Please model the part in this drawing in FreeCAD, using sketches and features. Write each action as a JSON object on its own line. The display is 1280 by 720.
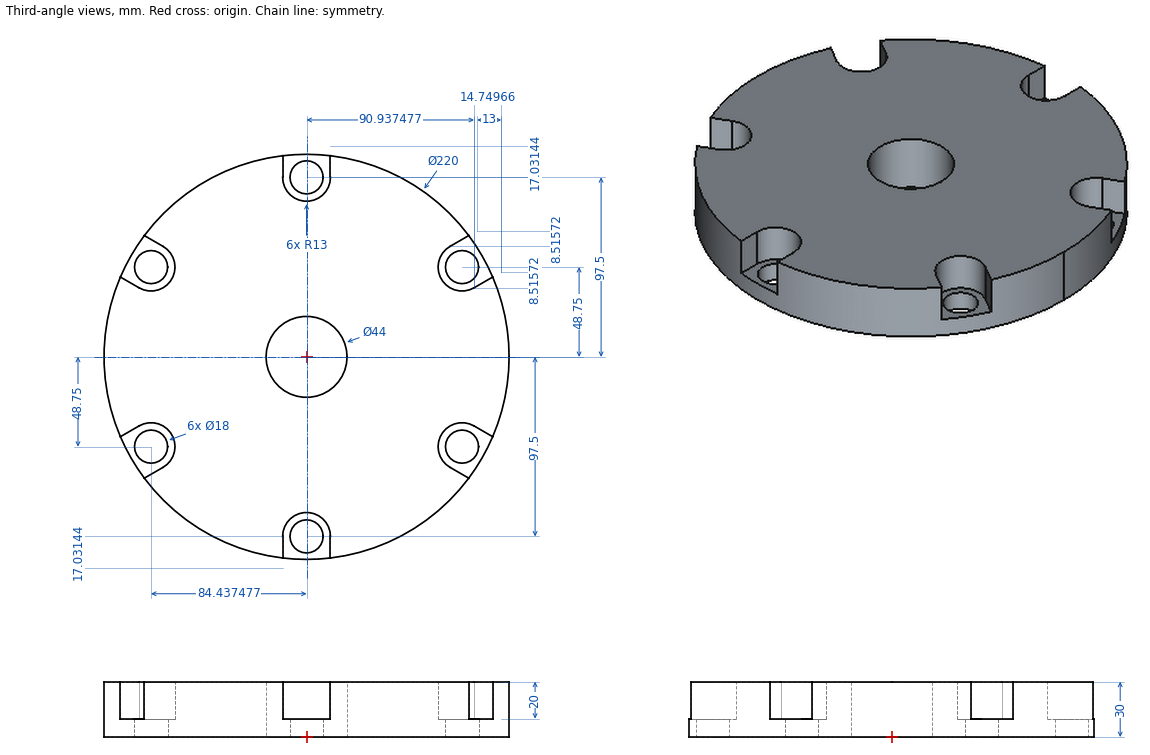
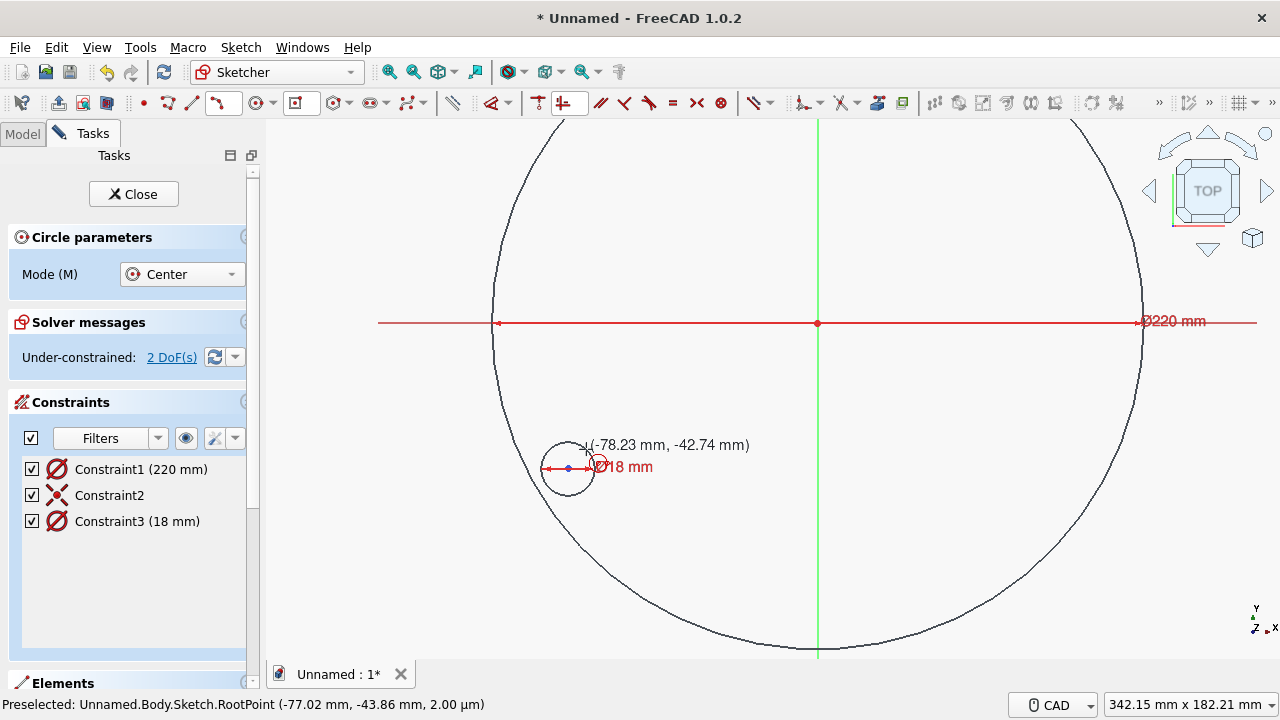
{"action": "left_click", "coordinate": [818, 612]}
{"action": "mouse_move", "coordinate": [837, 593]}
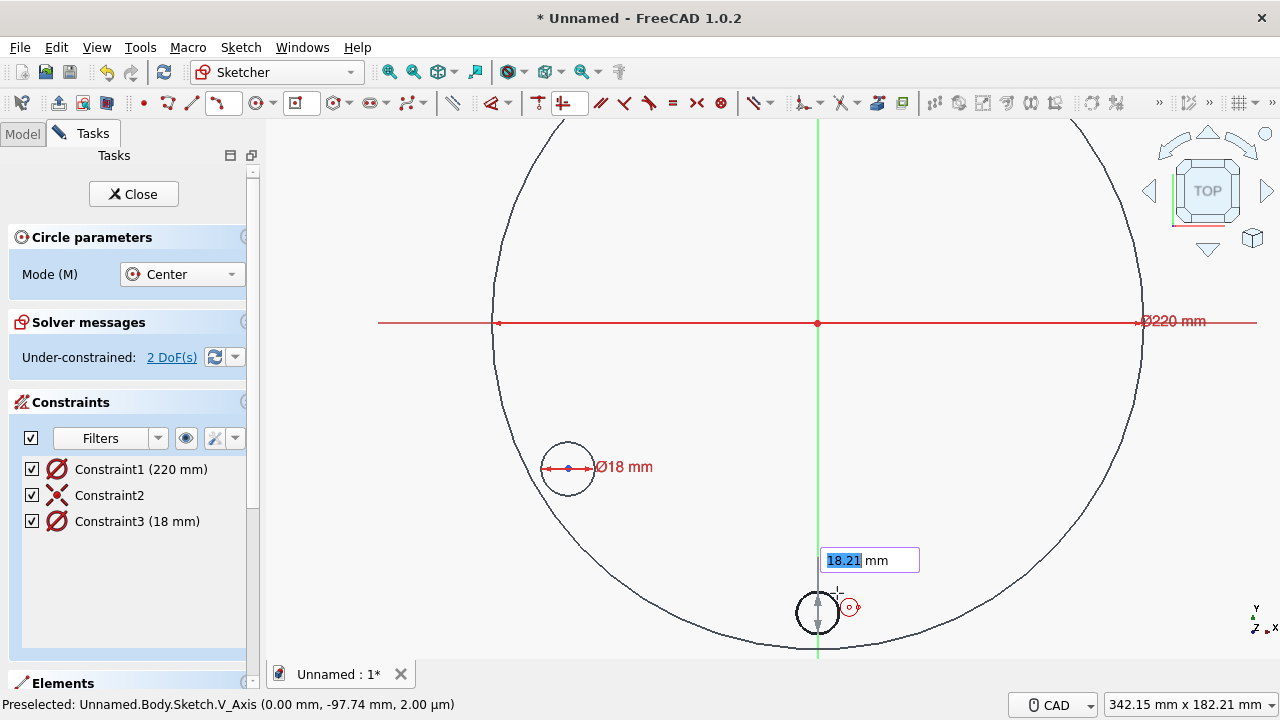
{"action": "type", "text": "18"}
{"action": "key", "text": "Return"}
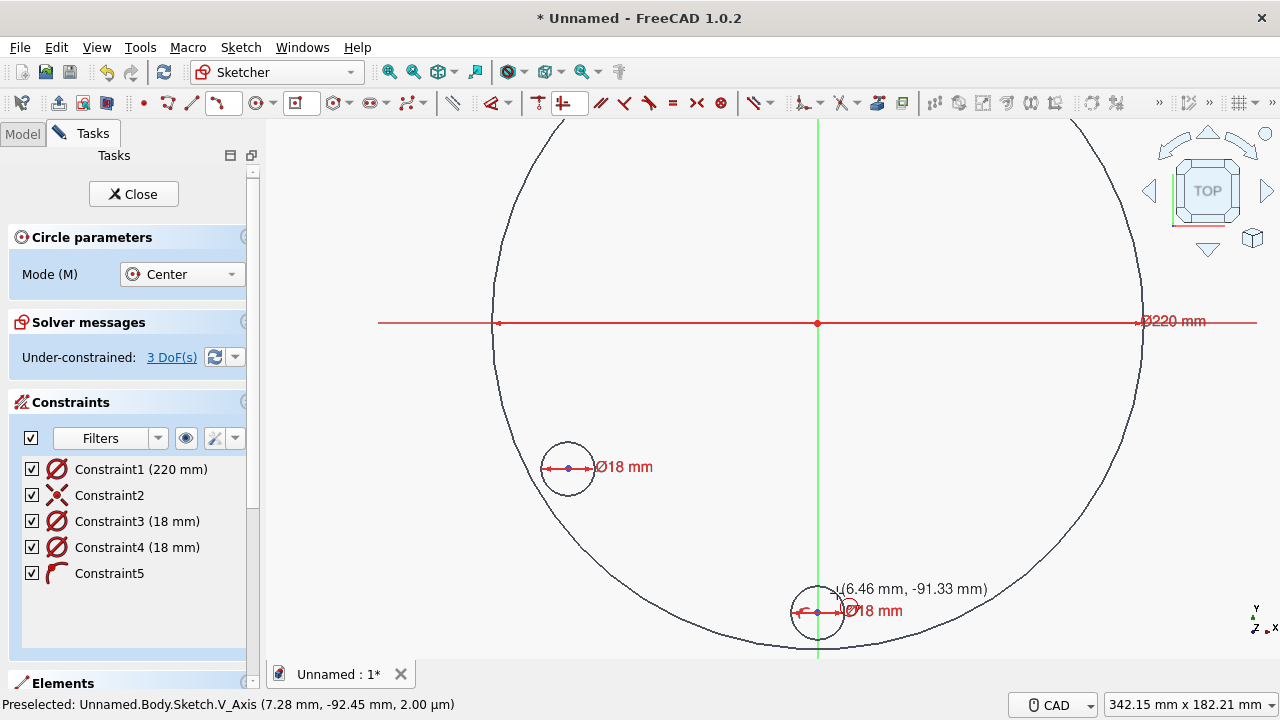
{"action": "left_click", "coordinate": [1068, 468]}
{"action": "mouse_move", "coordinate": [1087, 449]}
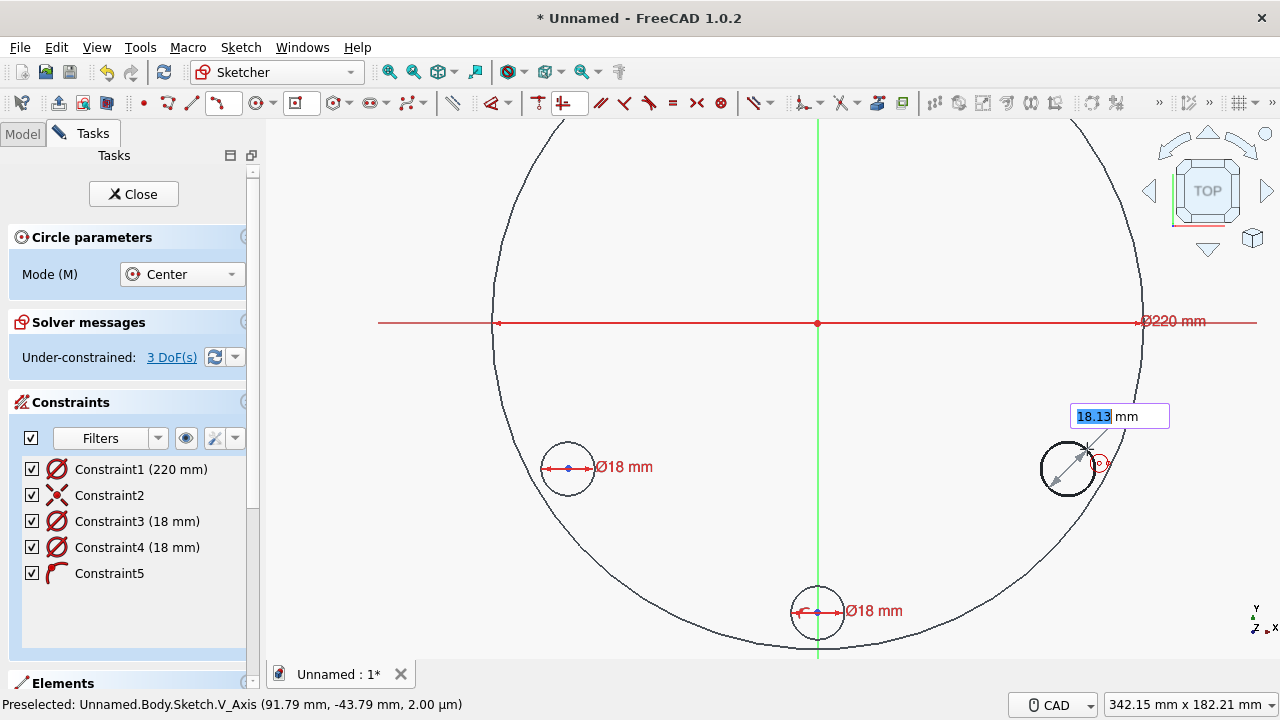
{"action": "type", "text": "18"}
{"action": "key", "text": "Return"}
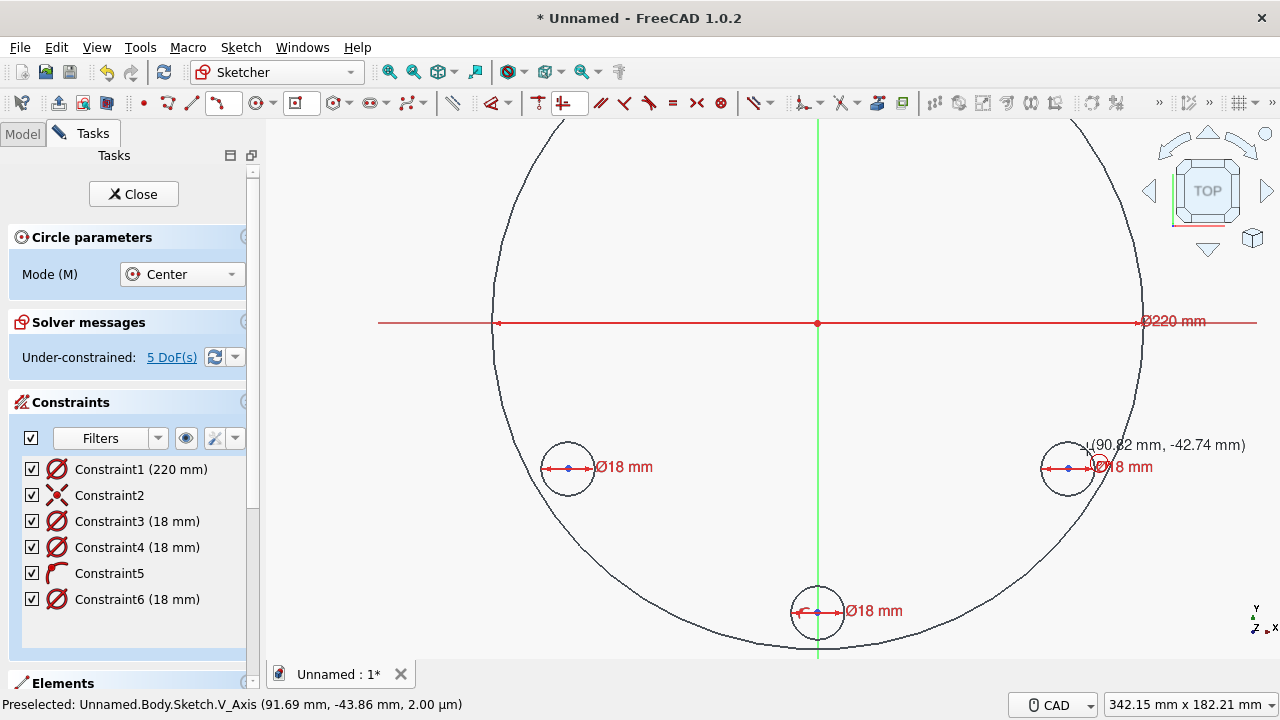
{"action": "left_click", "coordinate": [568, 179]}
{"action": "mouse_move", "coordinate": [586, 160]}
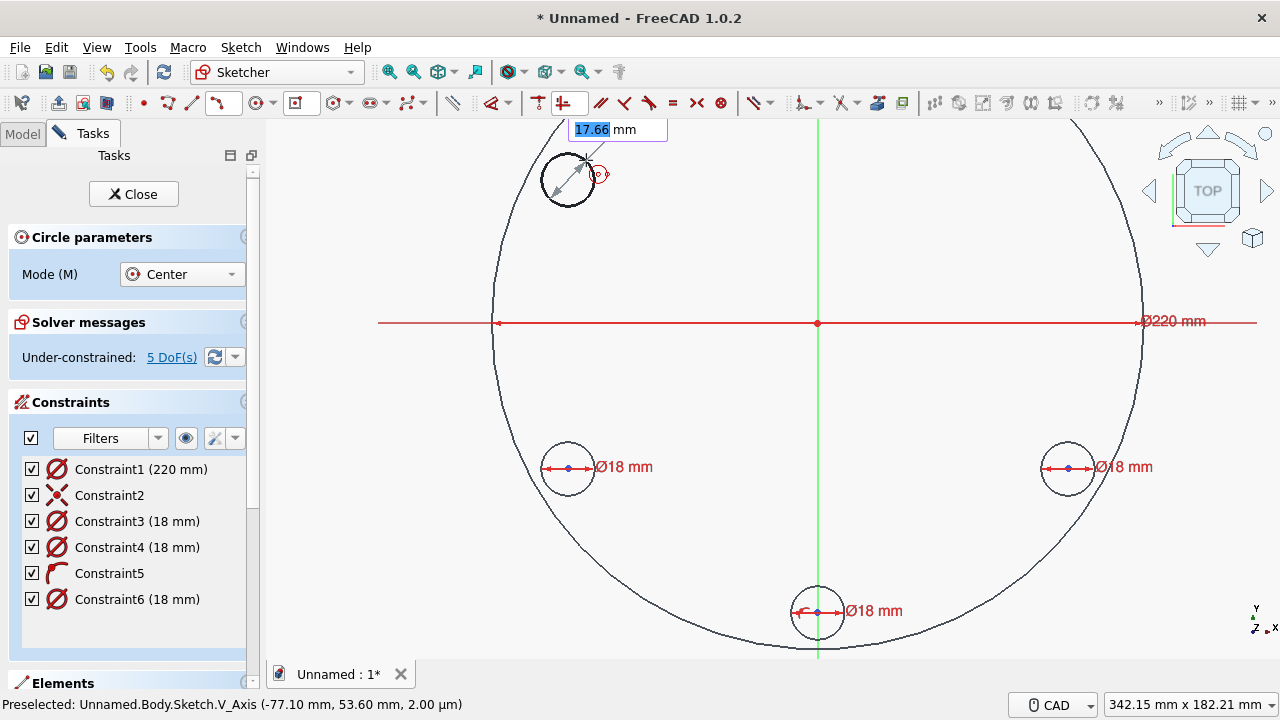
{"action": "type", "text": "18"}
{"action": "key", "text": "Return"}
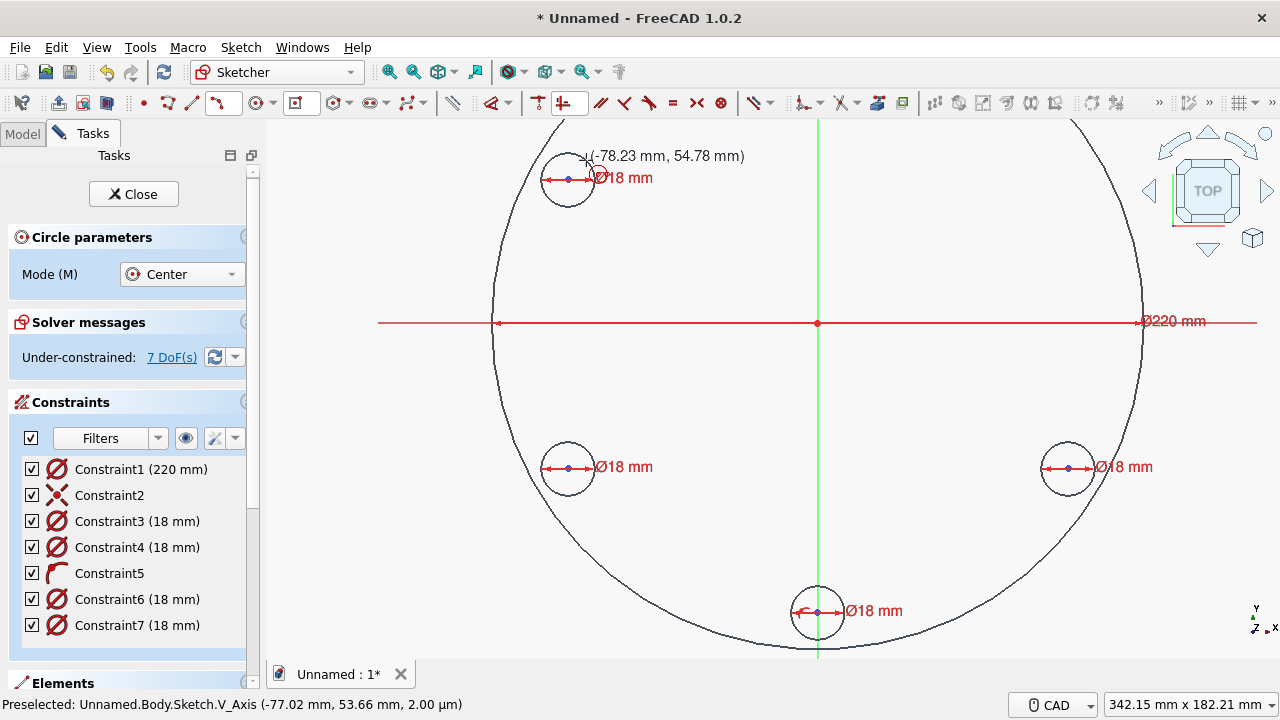
{"action": "left_click", "coordinate": [818, 323]}
{"action": "mouse_move", "coordinate": [864, 277]}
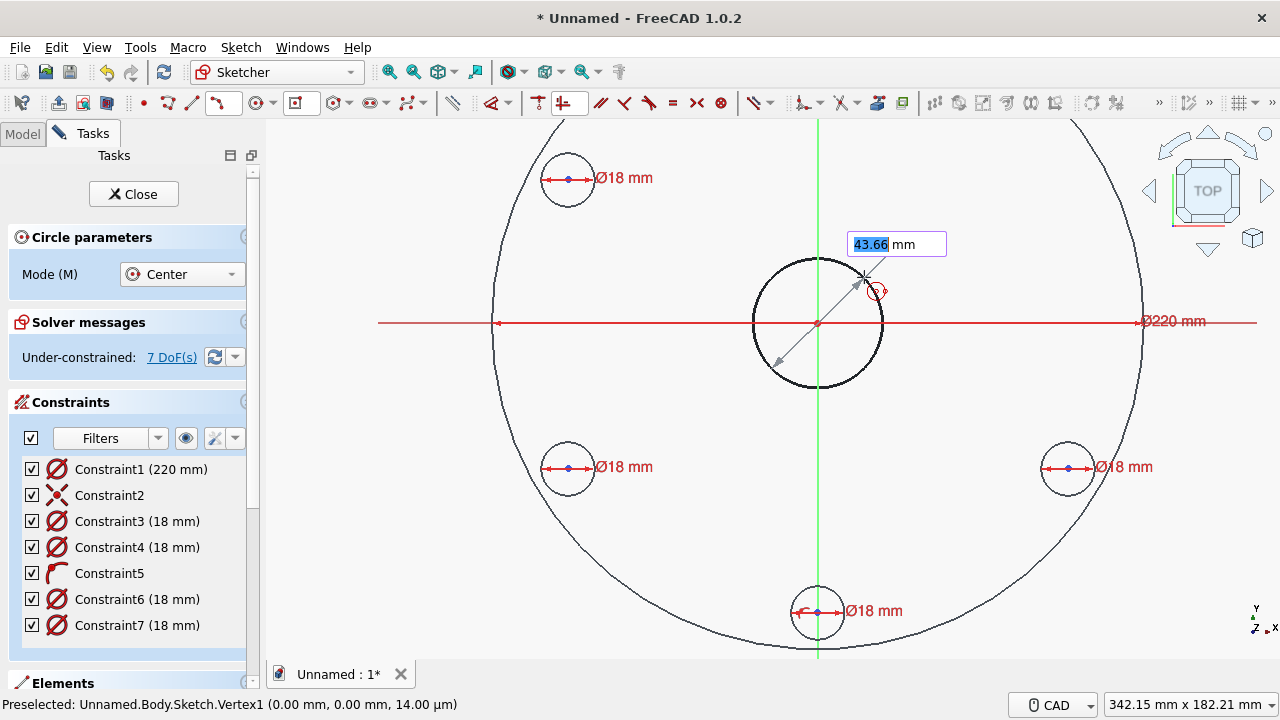
{"action": "type", "text": "44"}
{"action": "key", "text": "Return"}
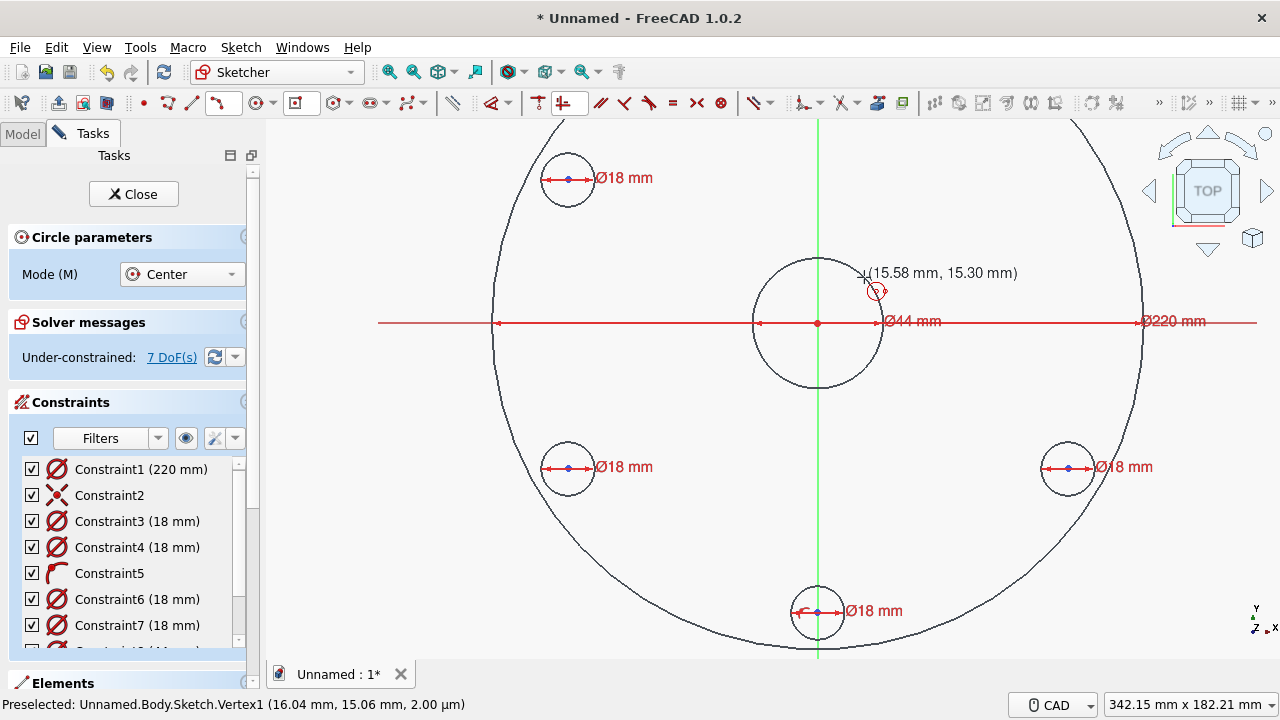
{"action": "left_click", "coordinate": [1068, 179]}
{"action": "mouse_move", "coordinate": [1049, 160]}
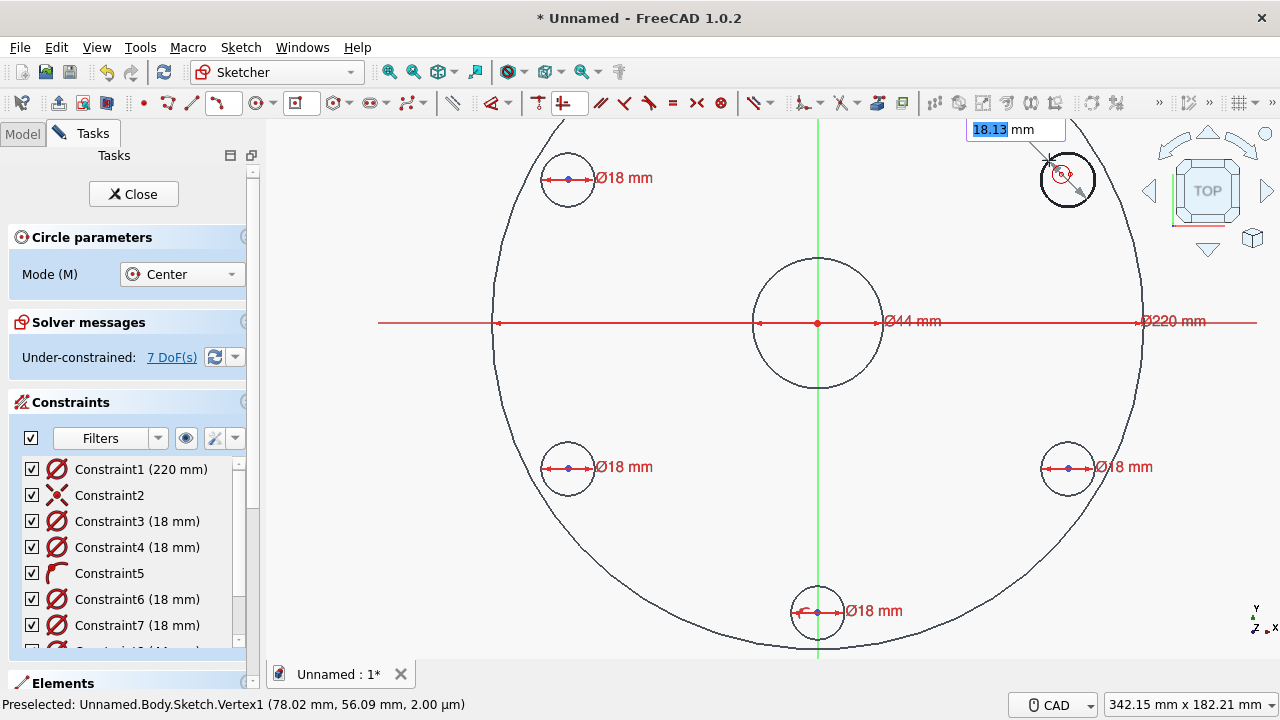
{"action": "type", "text": "18"}
{"action": "key", "text": "Return"}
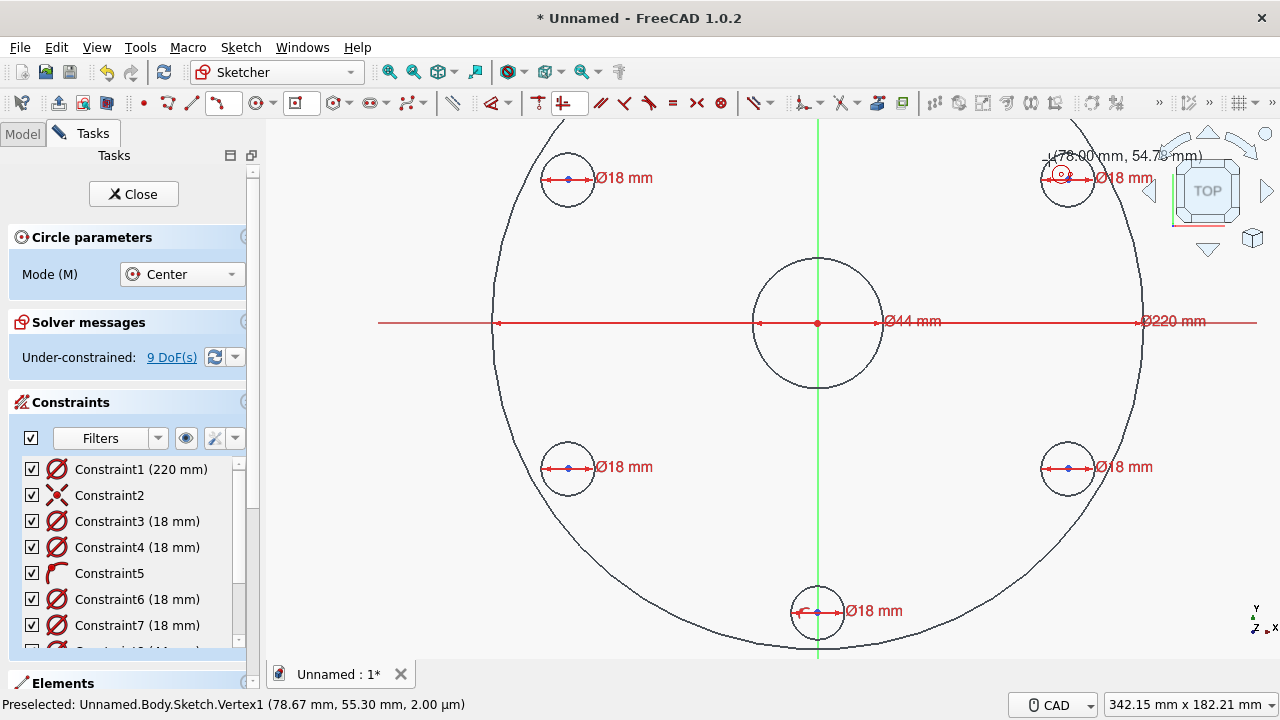
{"action": "scroll", "coordinate": [567, 469], "scroll_direction": "down", "scroll_amount": 3}